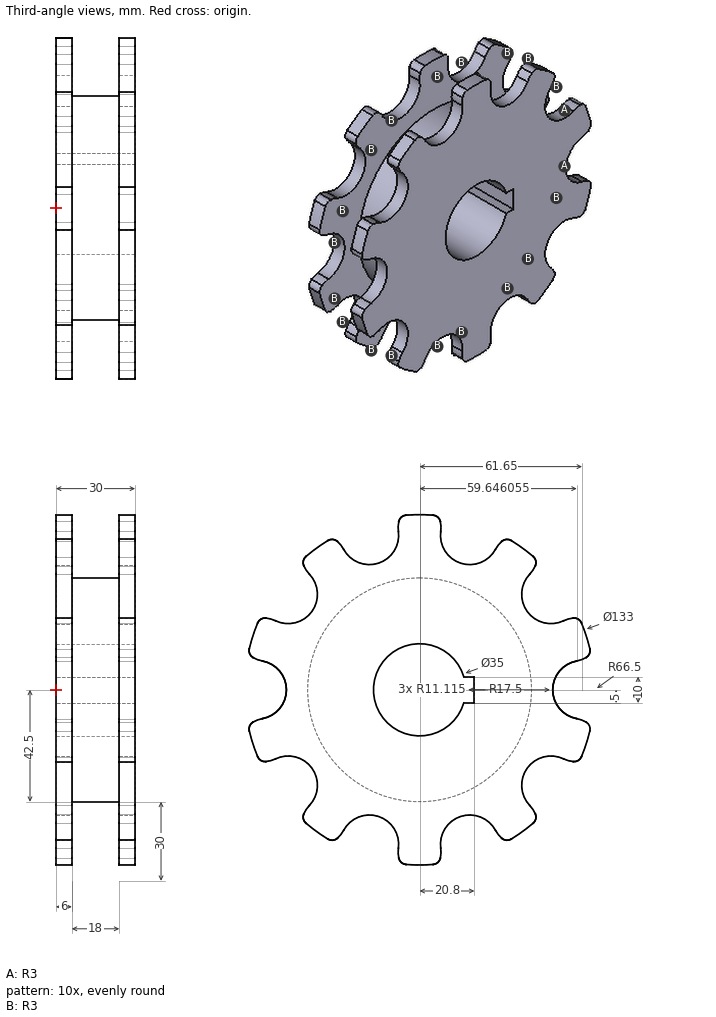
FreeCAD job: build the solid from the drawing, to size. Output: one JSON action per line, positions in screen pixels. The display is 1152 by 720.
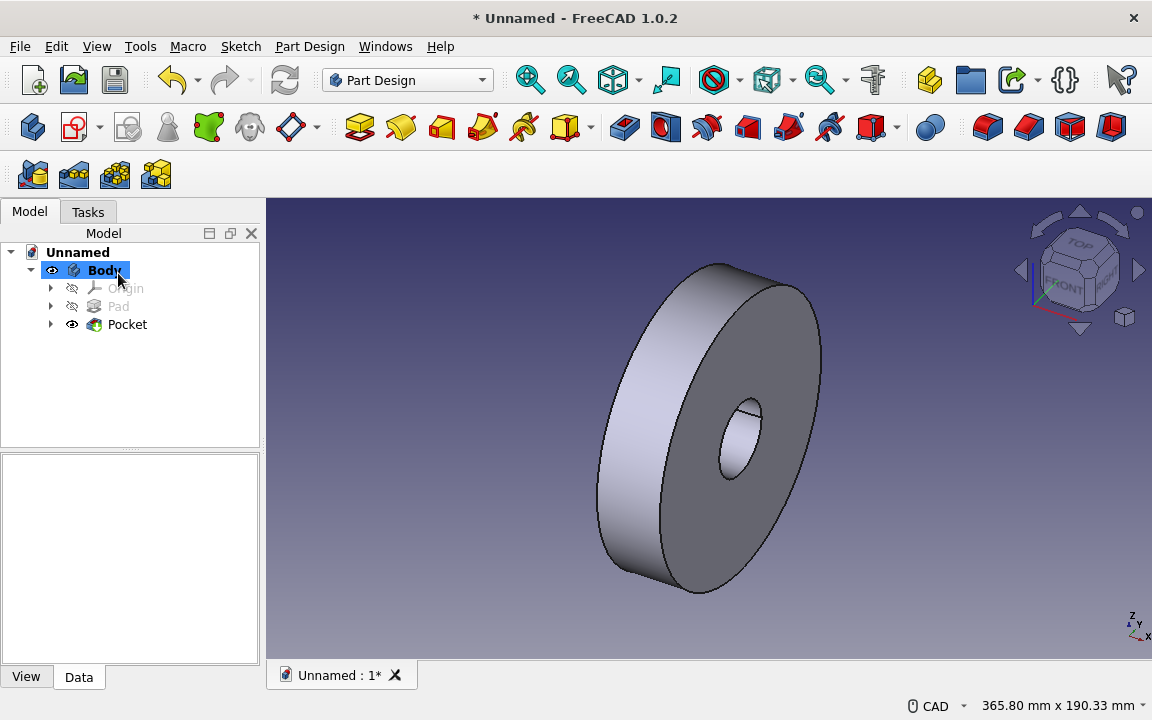
{"action": "left_click", "coordinate": [763, 490]}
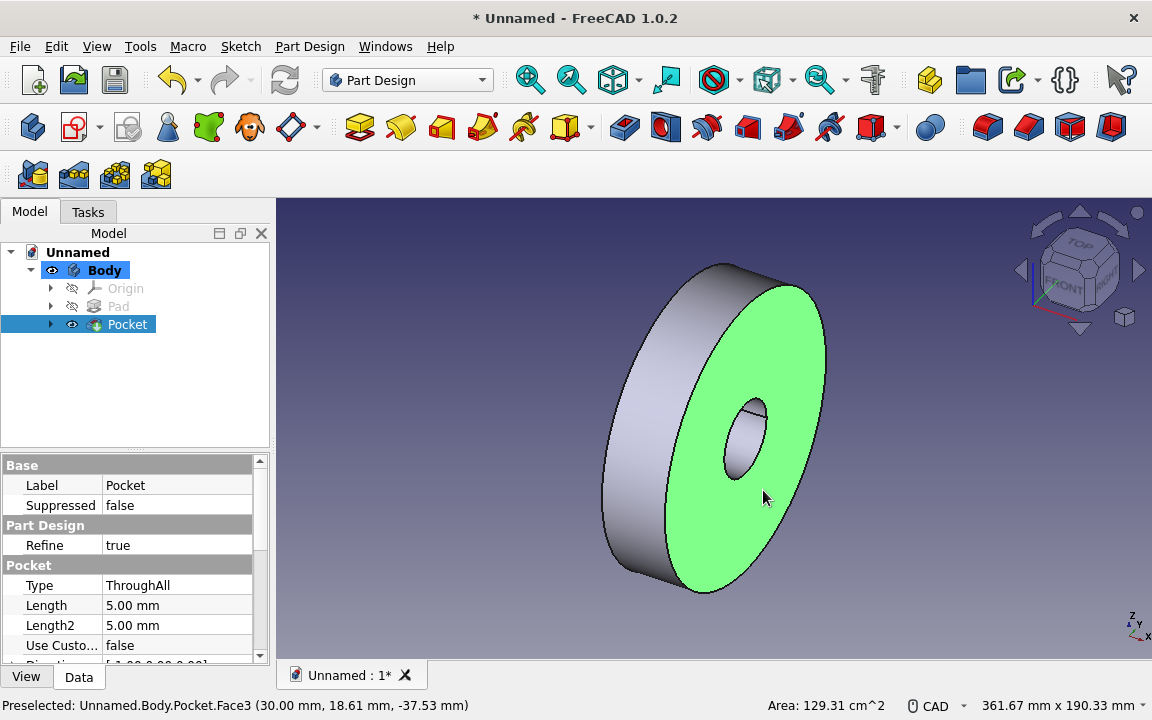
{"action": "left_click", "coordinate": [74, 128]}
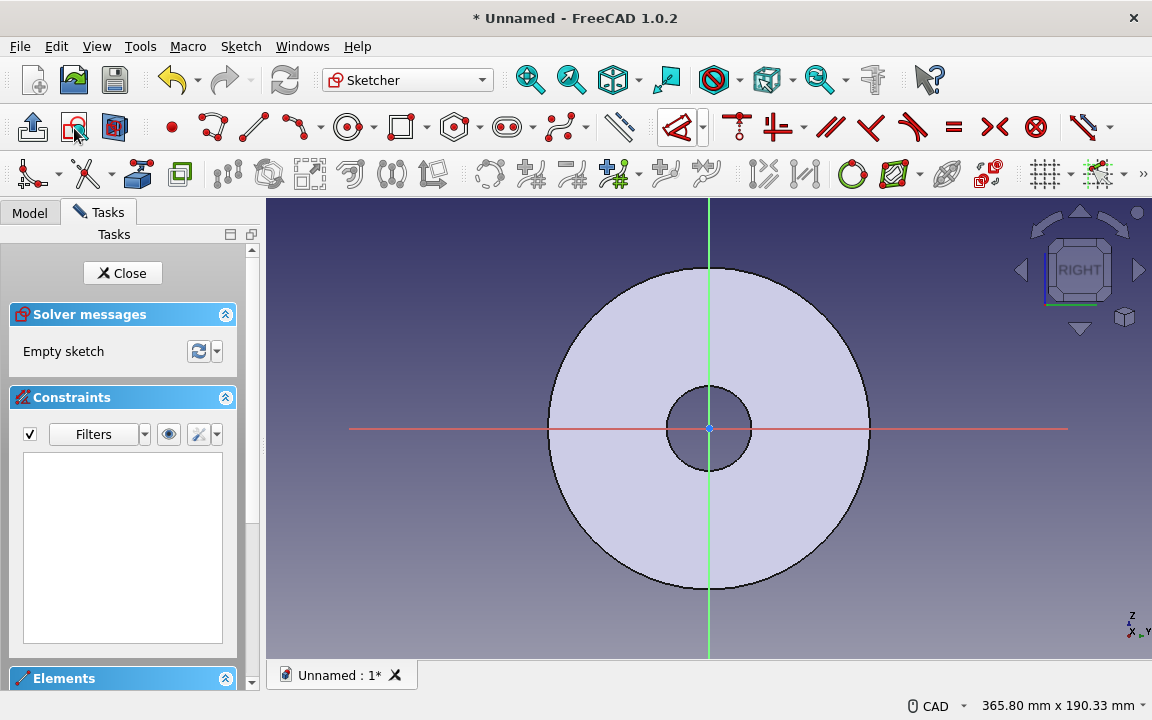
{"action": "scroll", "coordinate": [746, 428], "scroll_direction": "up", "scroll_amount": 11}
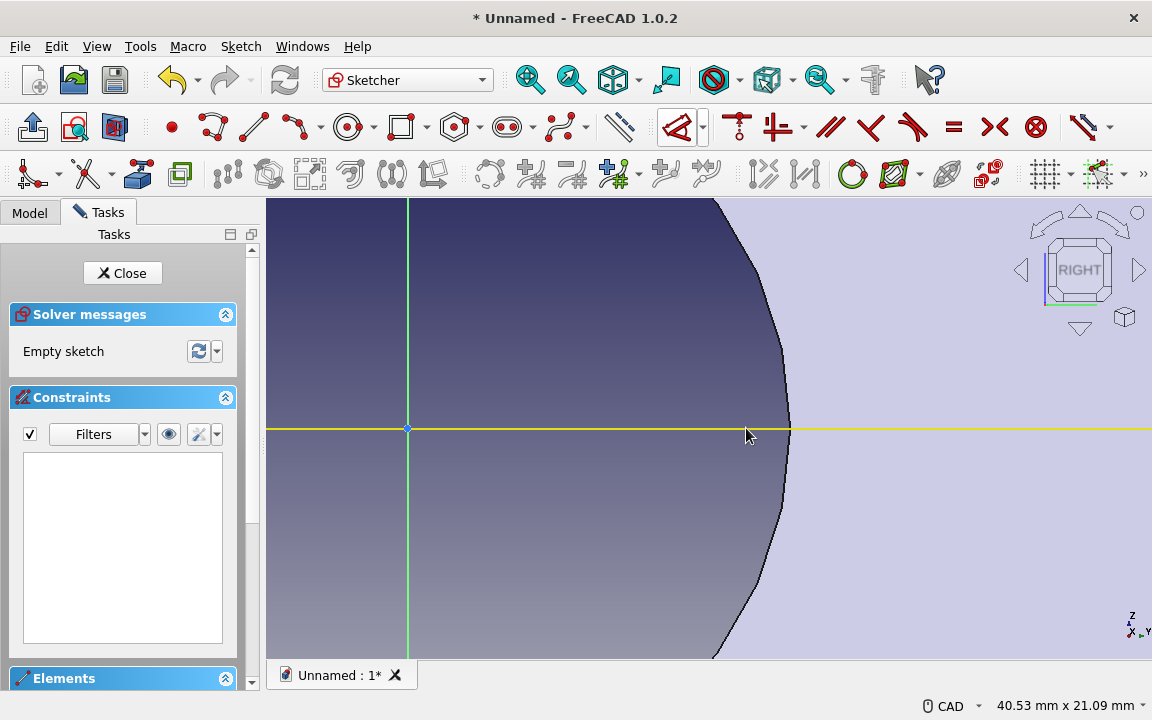
{"action": "left_click", "coordinate": [213, 128]}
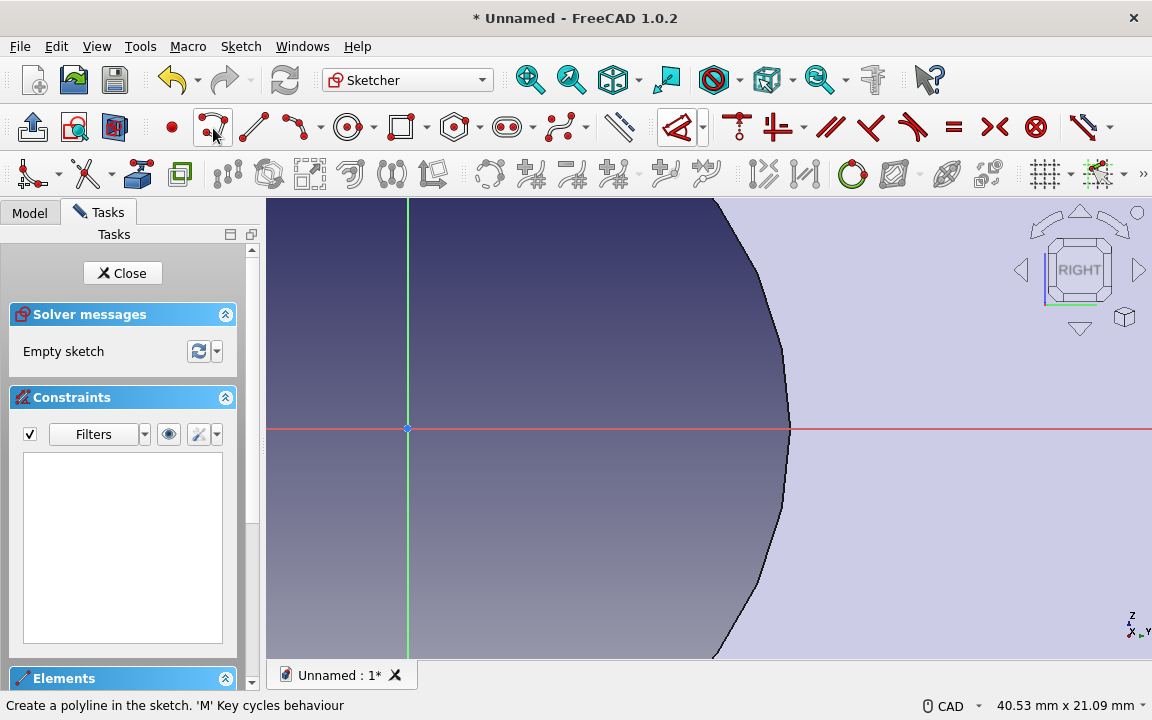
{"action": "left_click", "coordinate": [774, 538]}
{"action": "left_click", "coordinate": [862, 538]}
{"action": "left_click", "coordinate": [862, 319]}
{"action": "left_click", "coordinate": [774, 319]}
{"action": "right_click", "coordinate": [774, 319]}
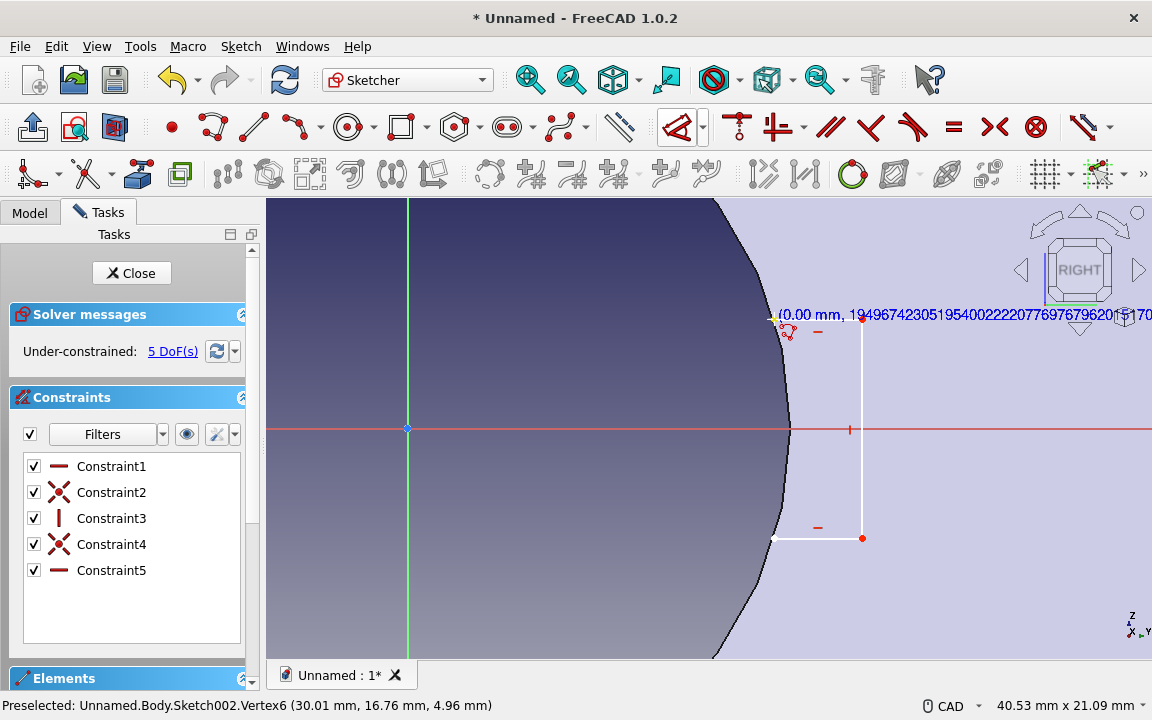
{"action": "left_click", "coordinate": [294, 128]}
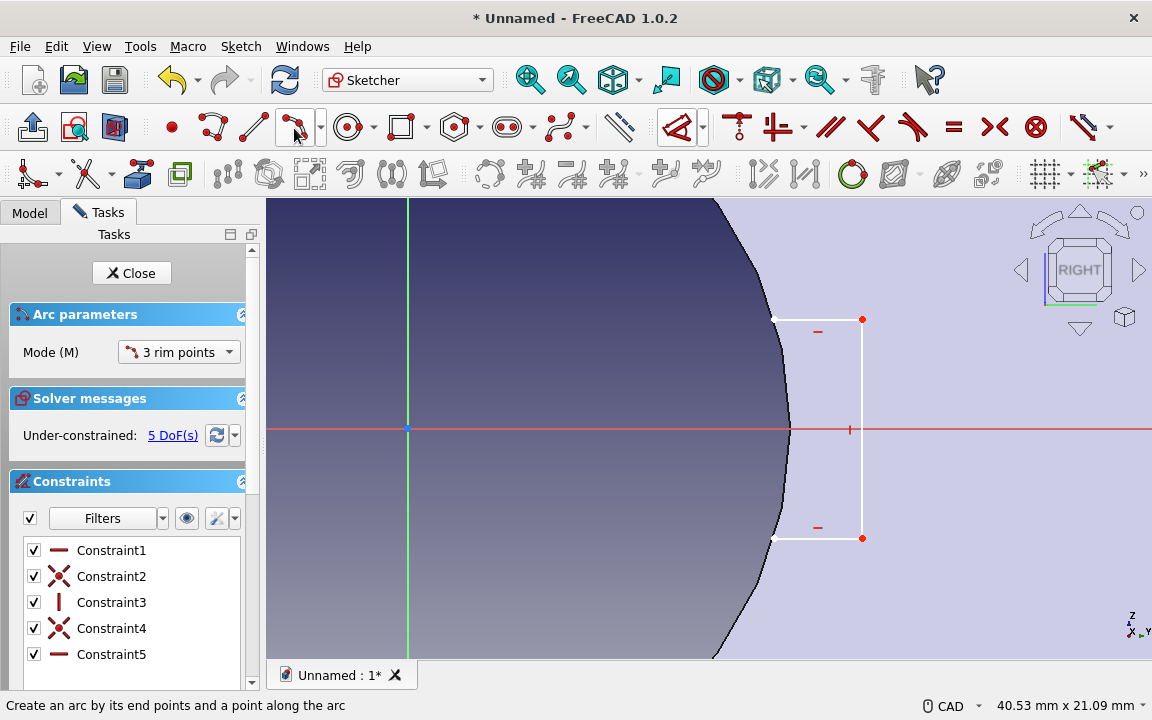
{"action": "left_click", "coordinate": [774, 320]}
{"action": "left_click", "coordinate": [774, 539]}
{"action": "left_click", "coordinate": [790, 451]}
{"action": "key", "text": "Escape"}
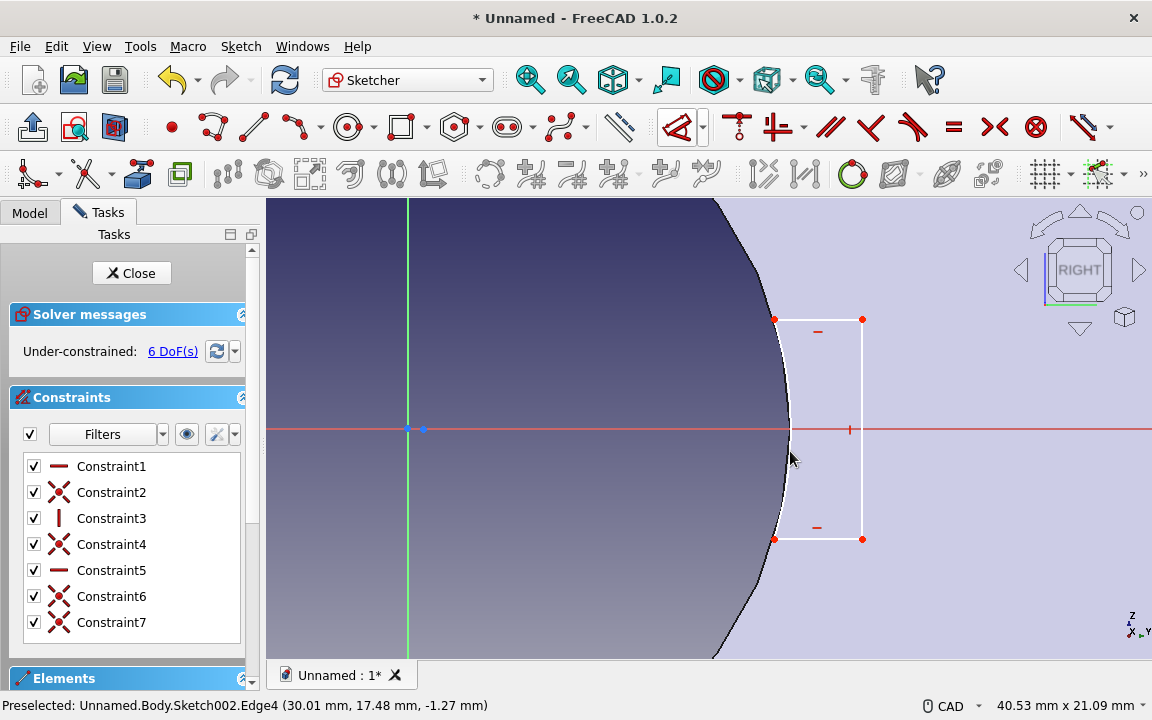
{"action": "left_click_drag", "start_coordinate": [398, 418], "coordinate": [433, 439]}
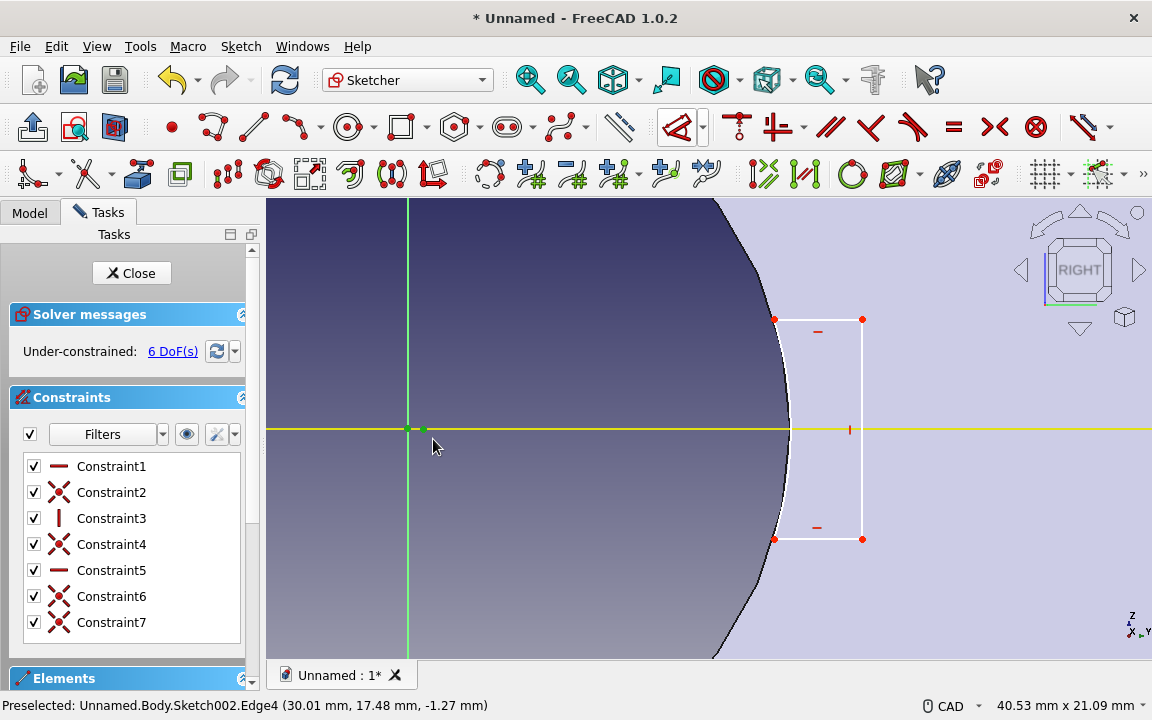
{"action": "left_click", "coordinate": [737, 128]}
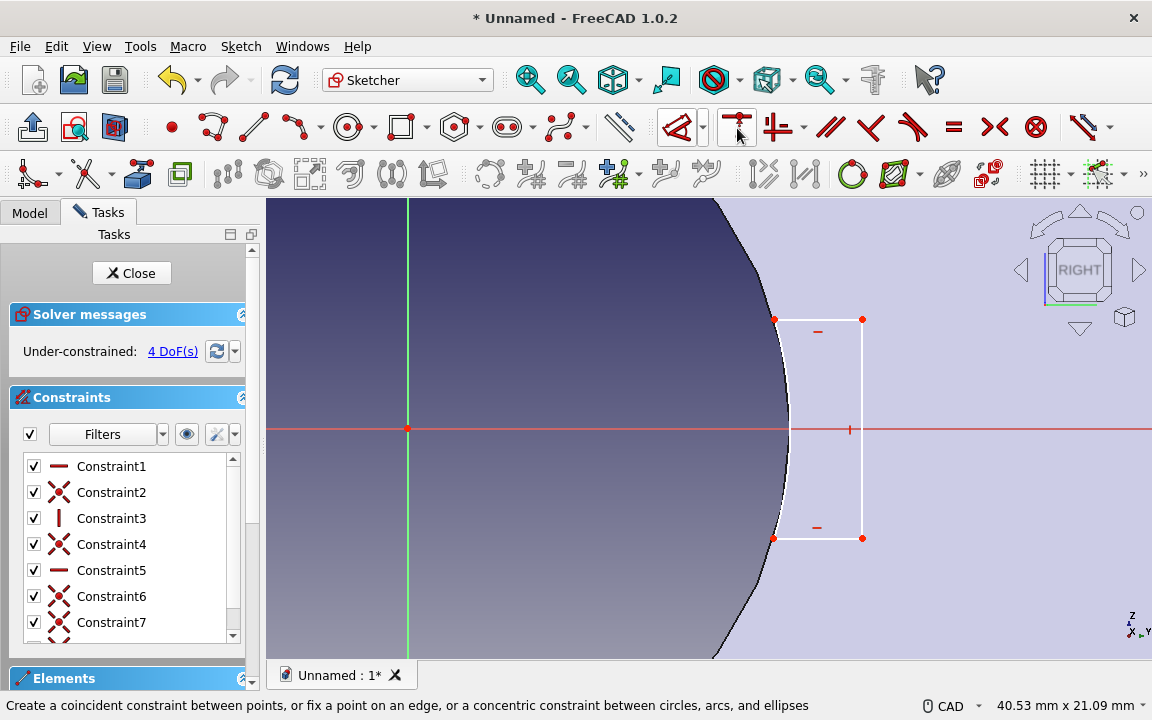
{"action": "left_click", "coordinate": [676, 128]}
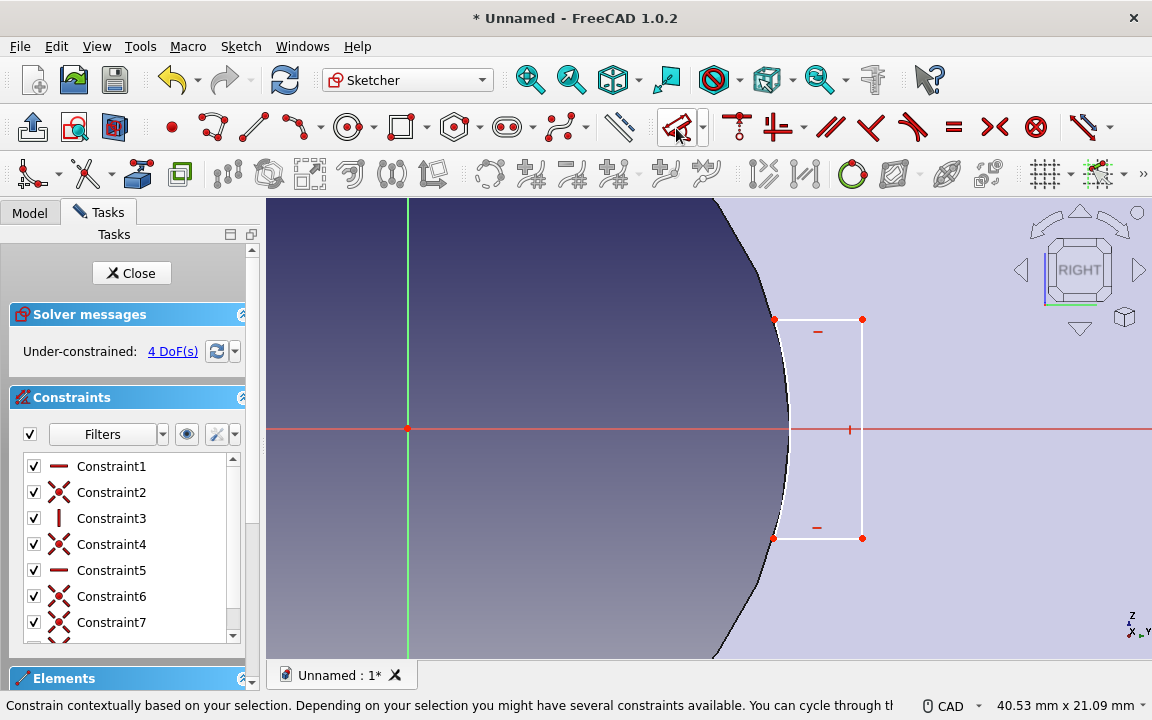
{"action": "left_click", "coordinate": [788, 474]}
{"action": "left_click", "coordinate": [820, 478]}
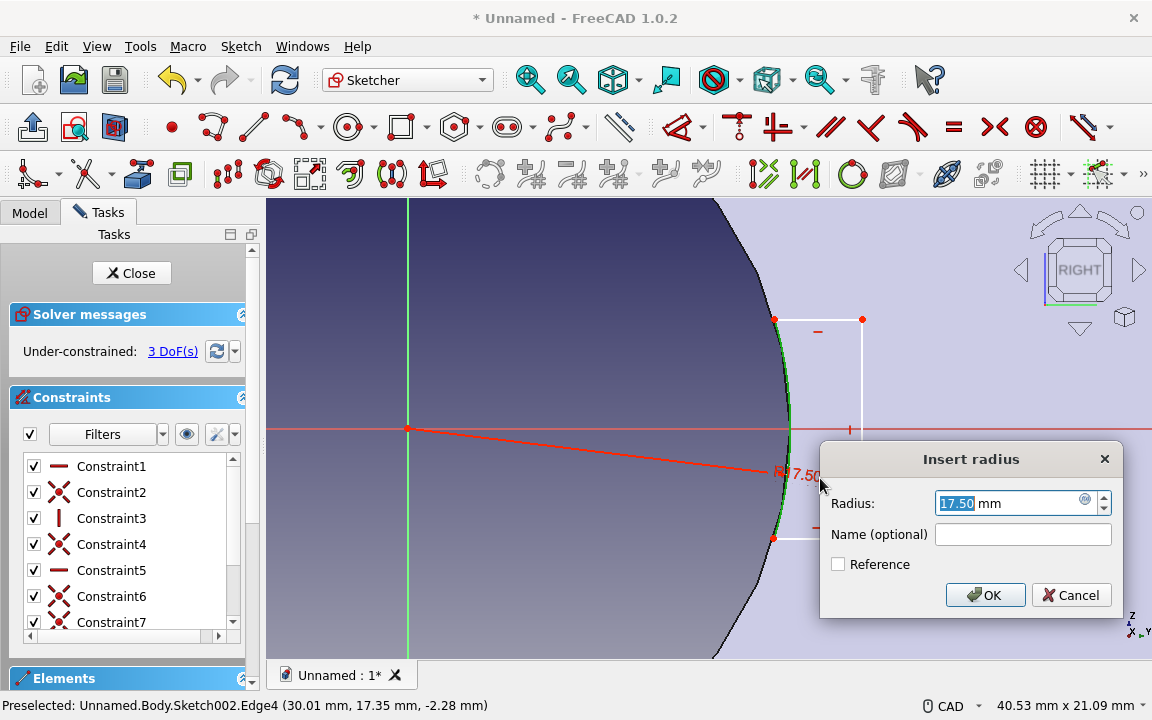
{"action": "type", "text": "17.5"}
{"action": "key", "text": "Return"}